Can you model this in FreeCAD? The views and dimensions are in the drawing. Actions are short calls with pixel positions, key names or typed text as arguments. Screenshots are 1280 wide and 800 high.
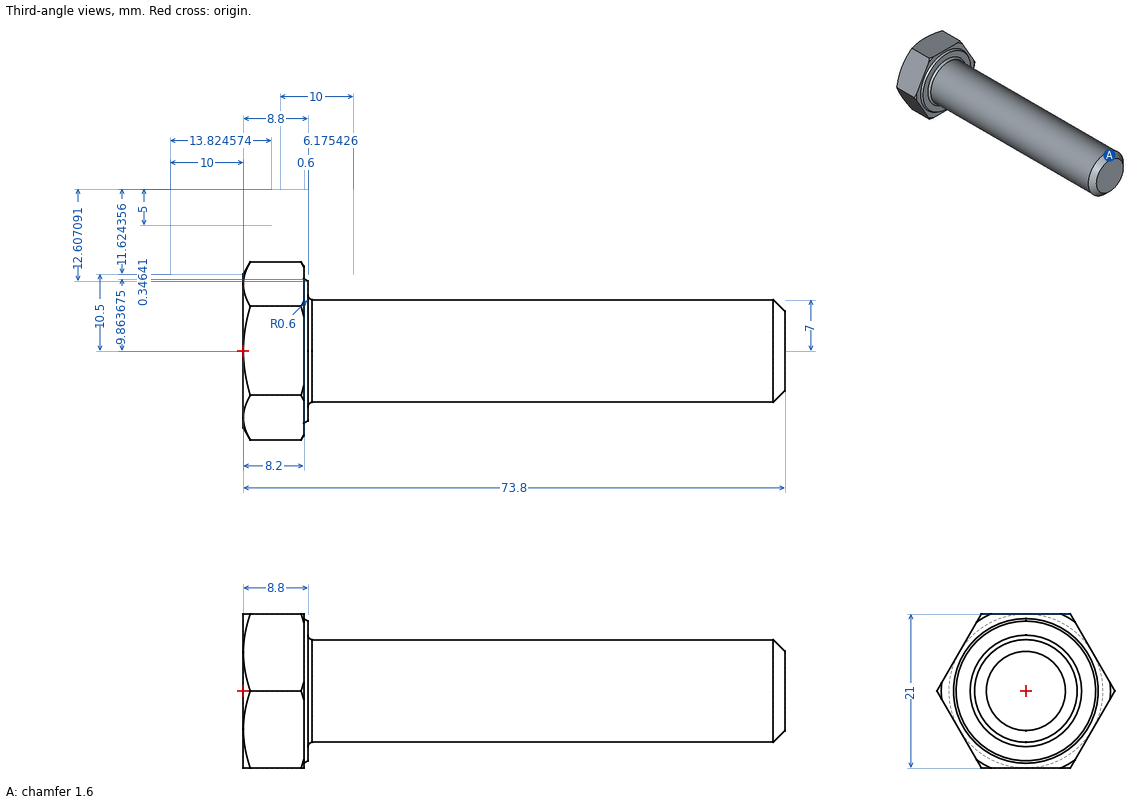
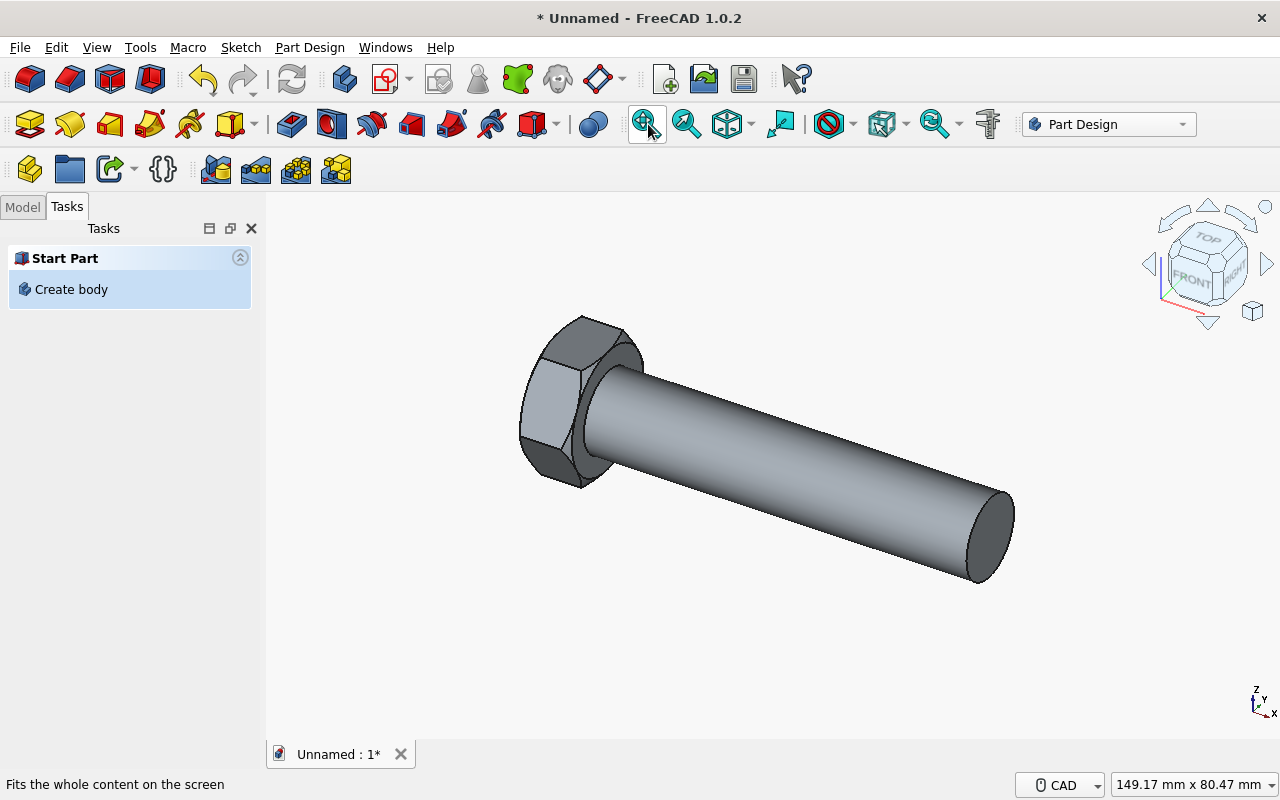
click(386, 80)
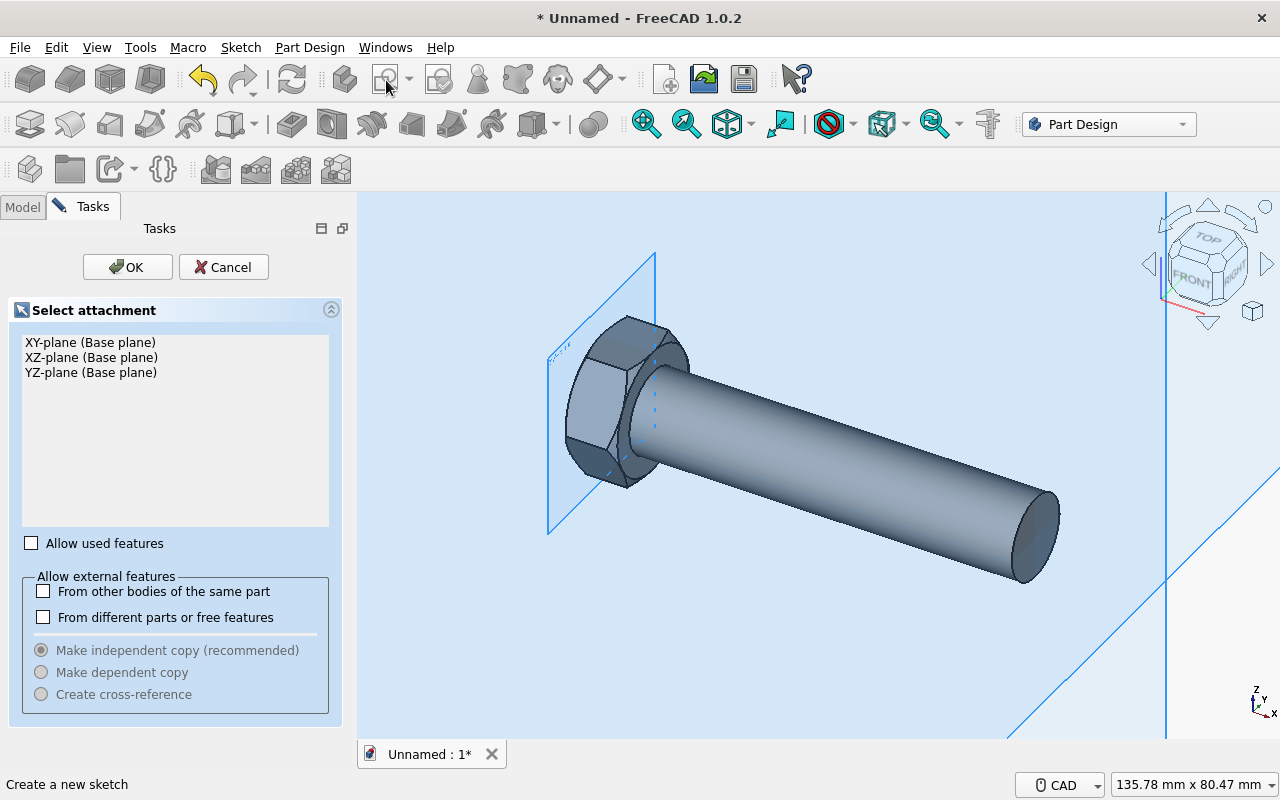
click(82, 342)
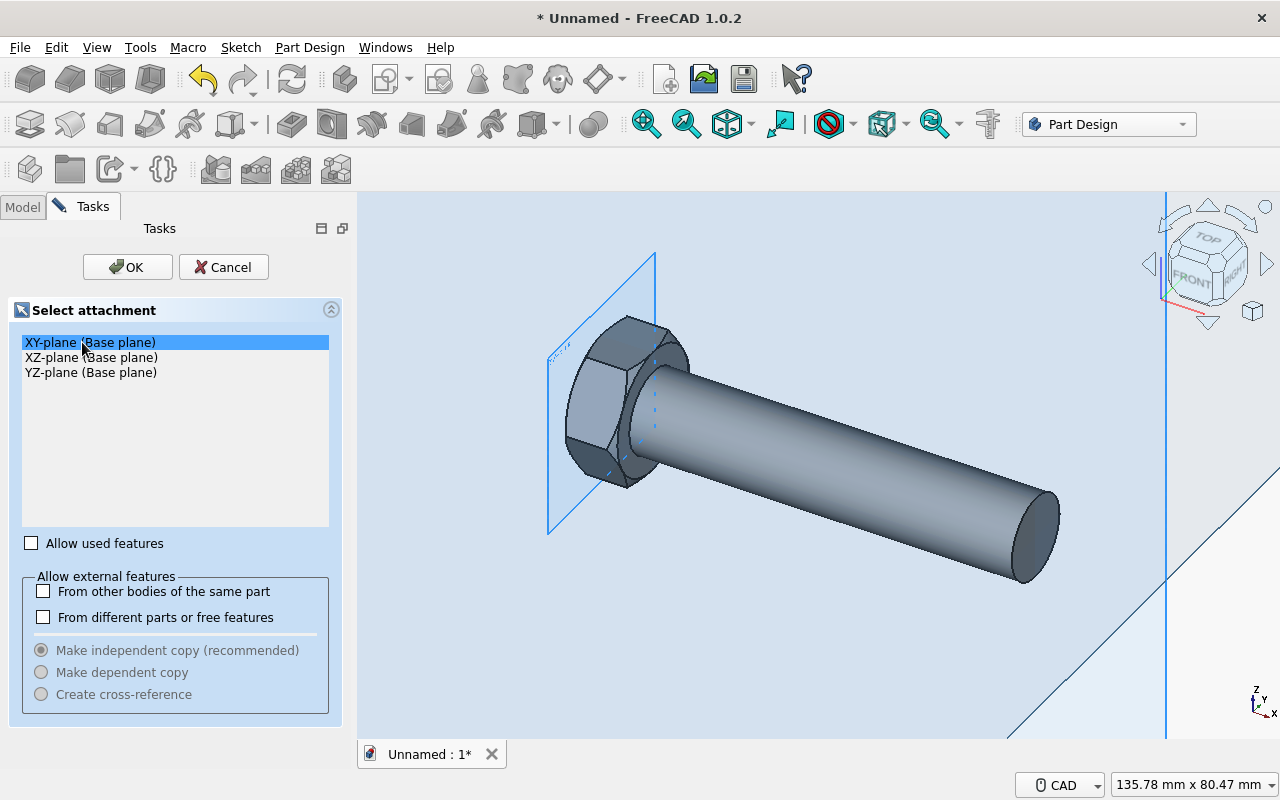
click(128, 267)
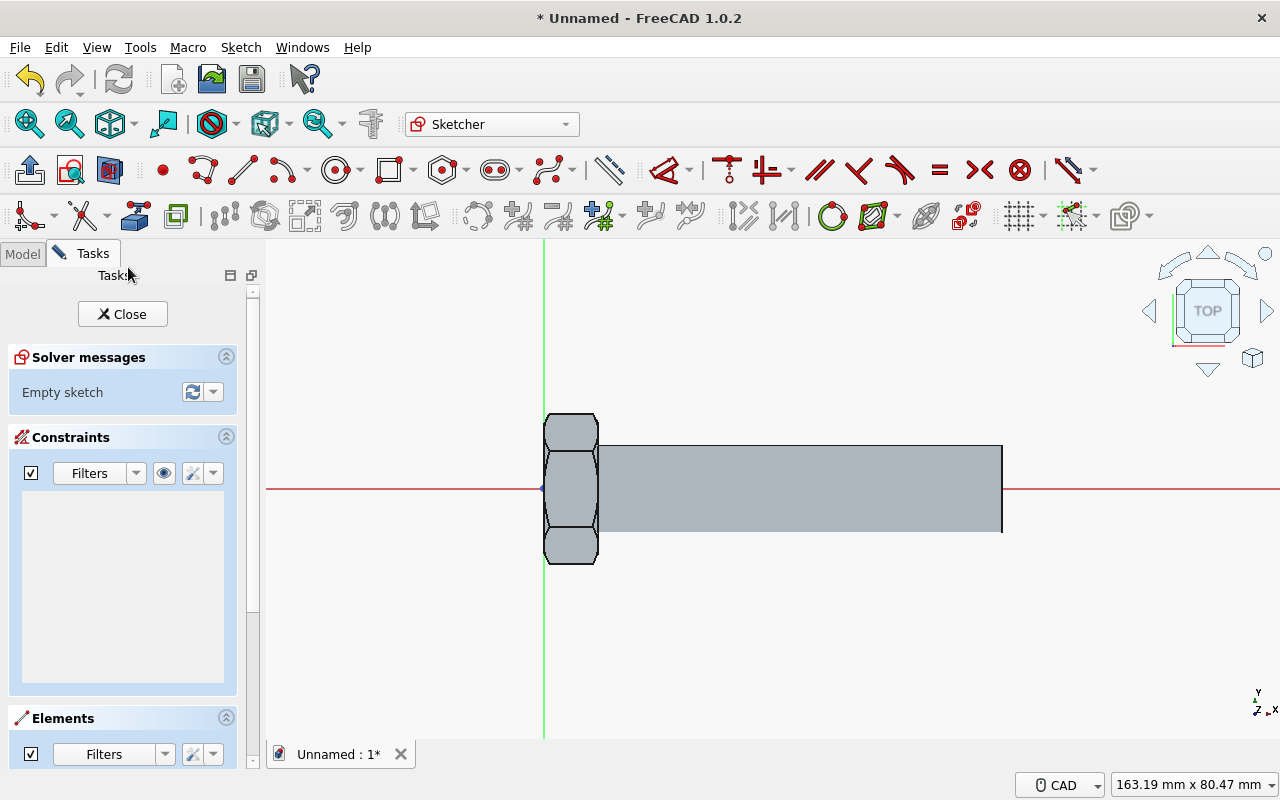
click(110, 170)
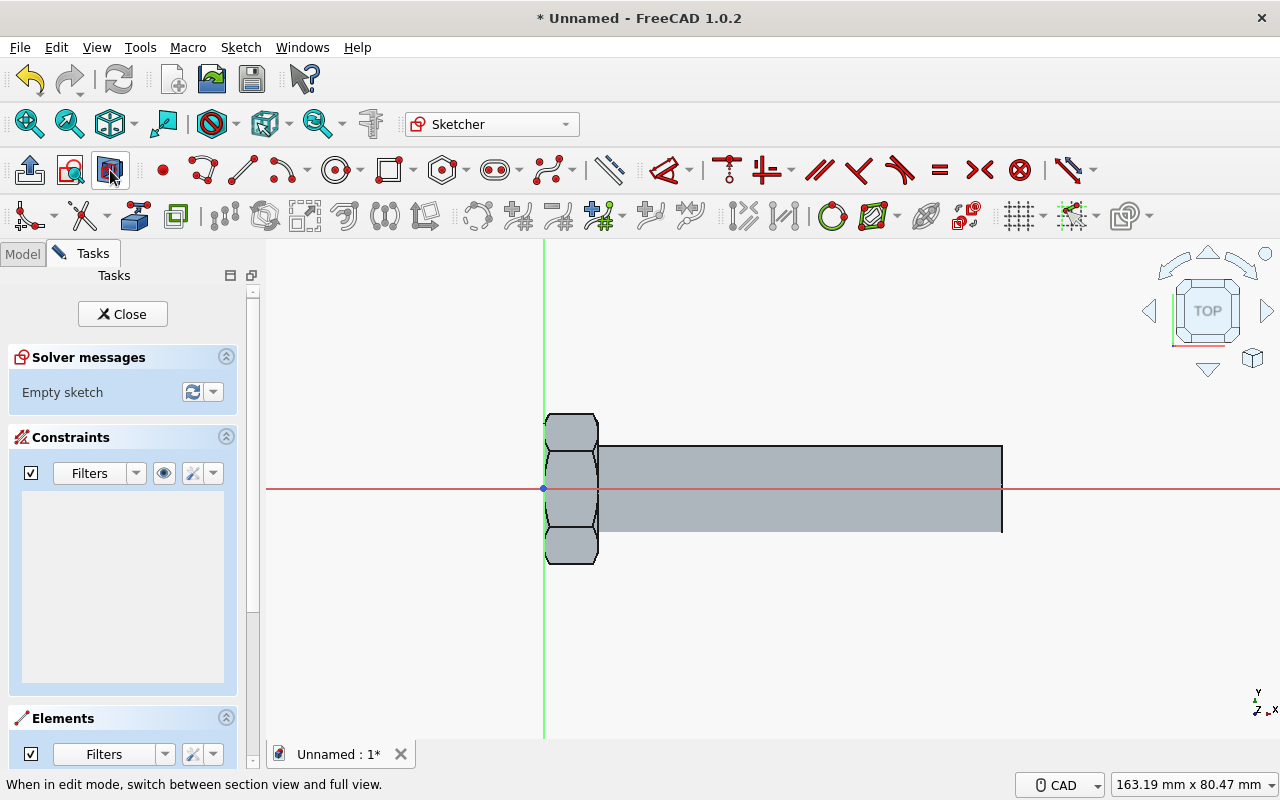
scroll(462, 364, up, 4)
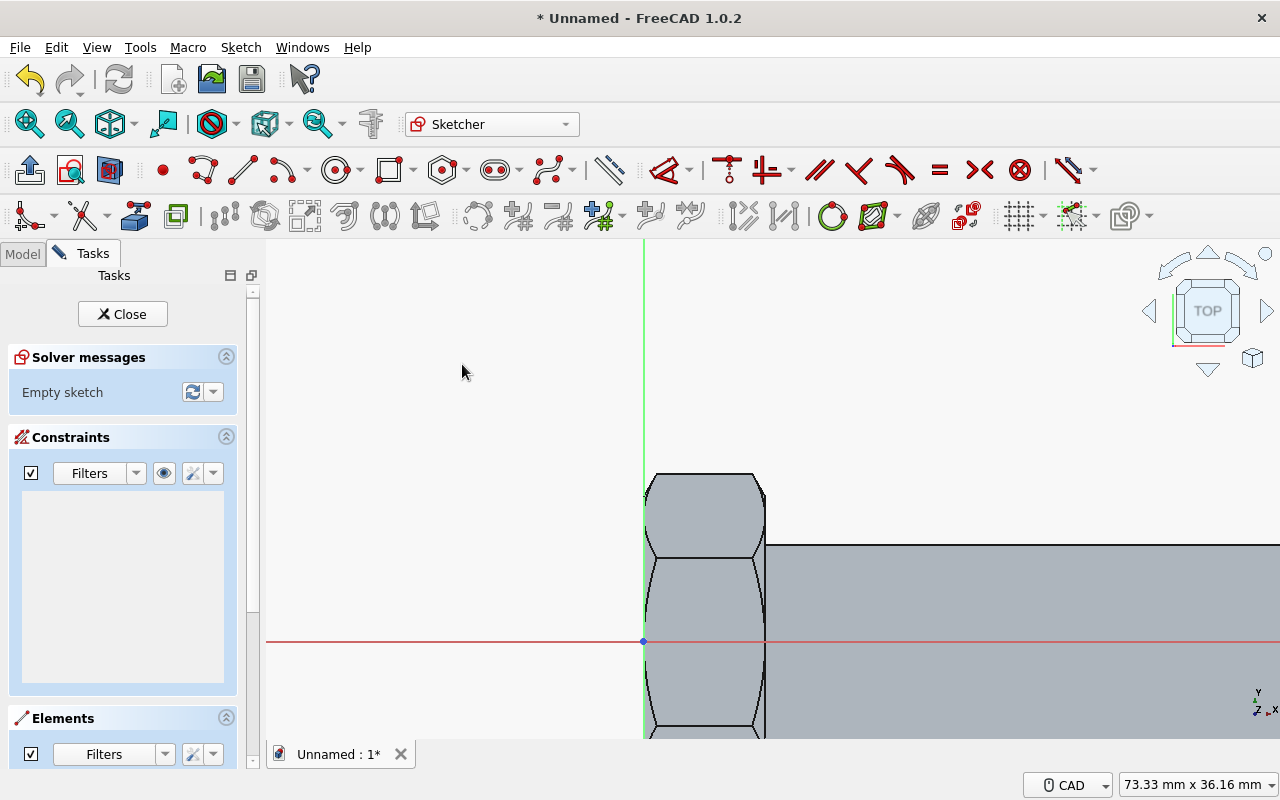
click(204, 170)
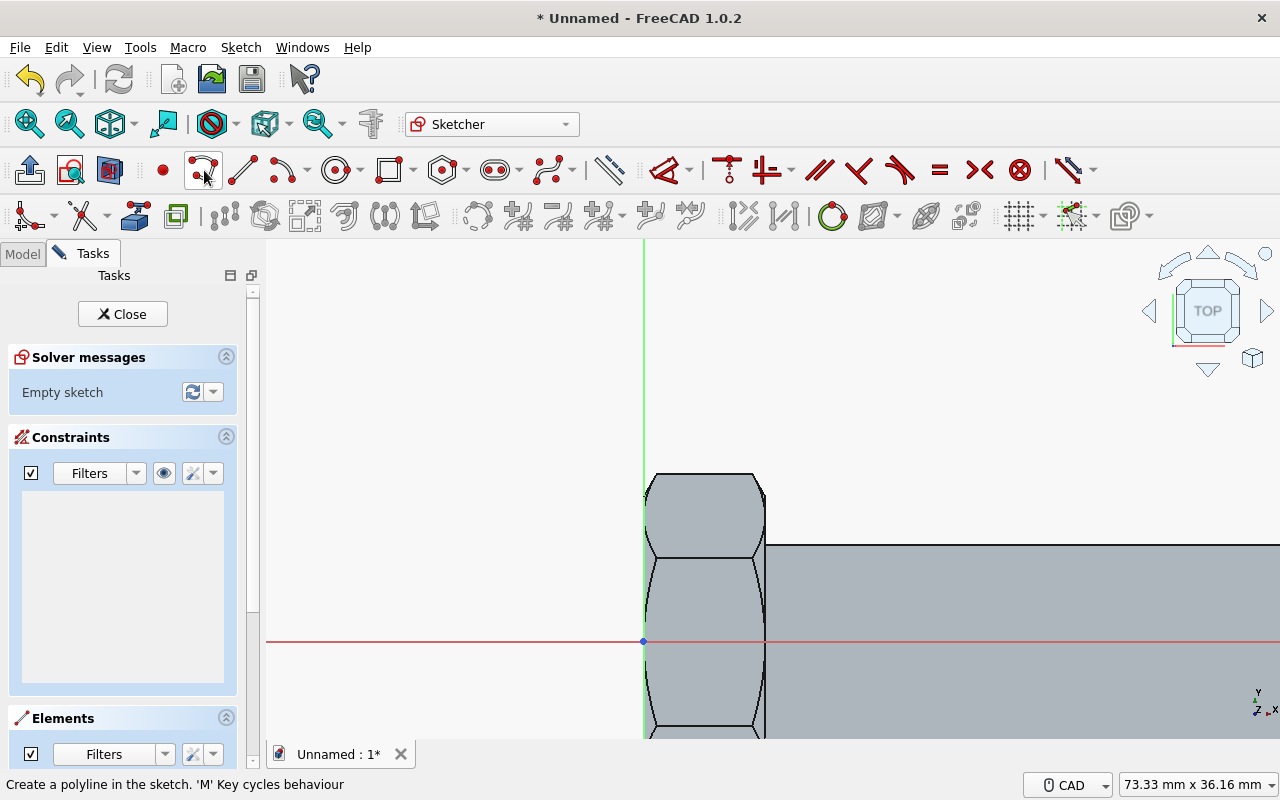
click(757, 505)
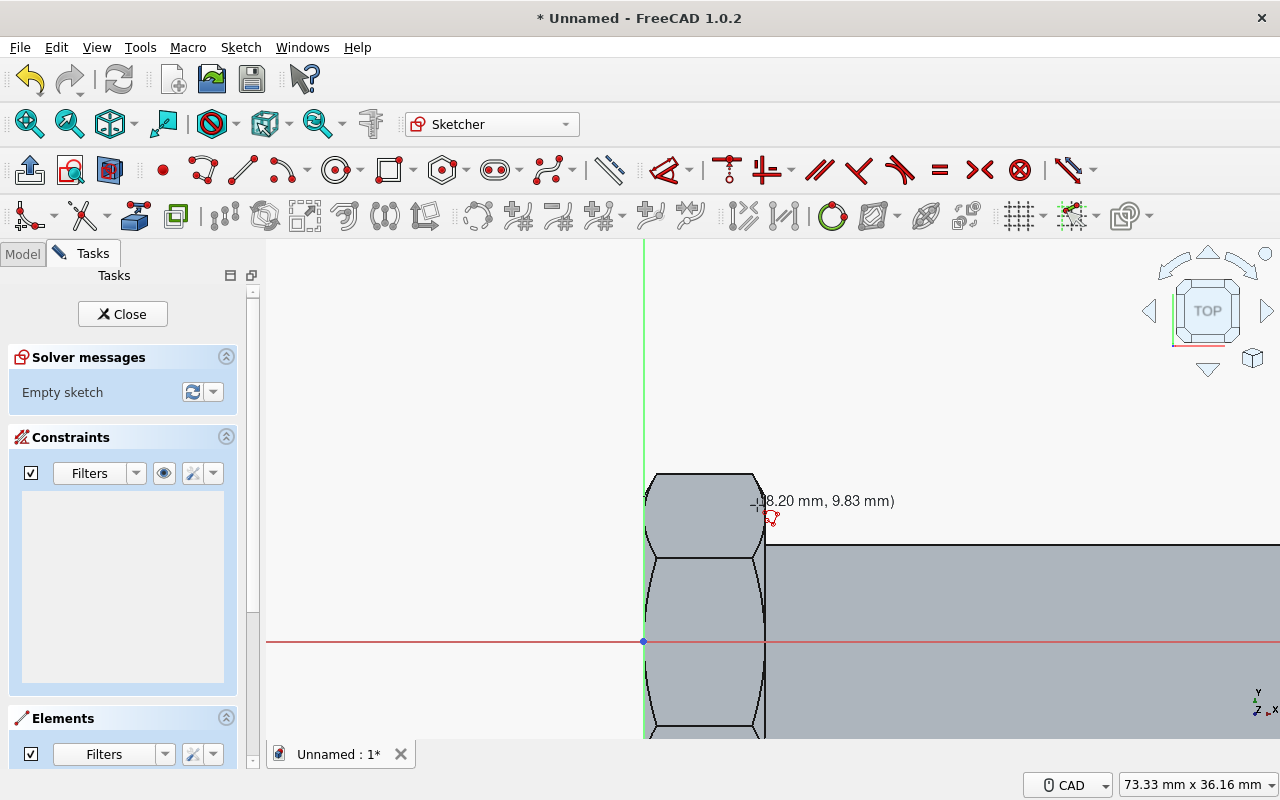
scroll(765, 510, up, 3)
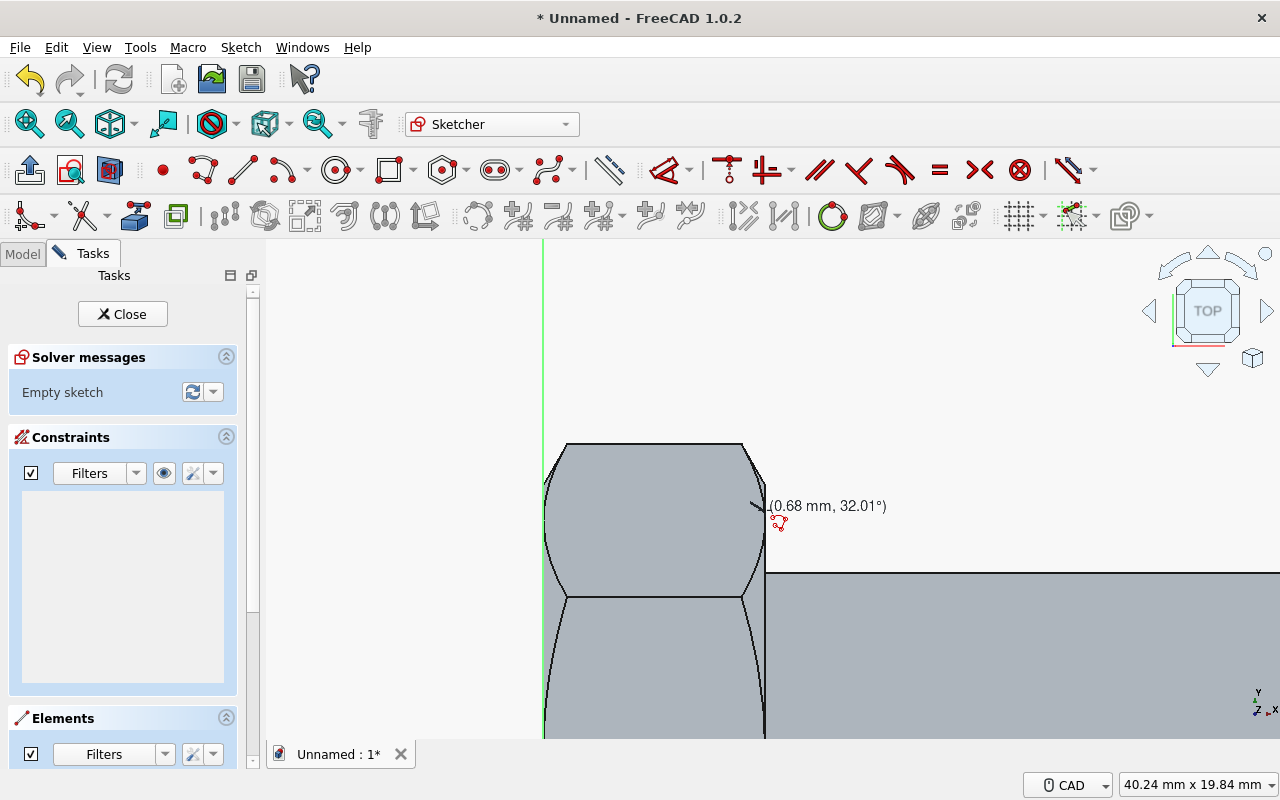
click(765, 510)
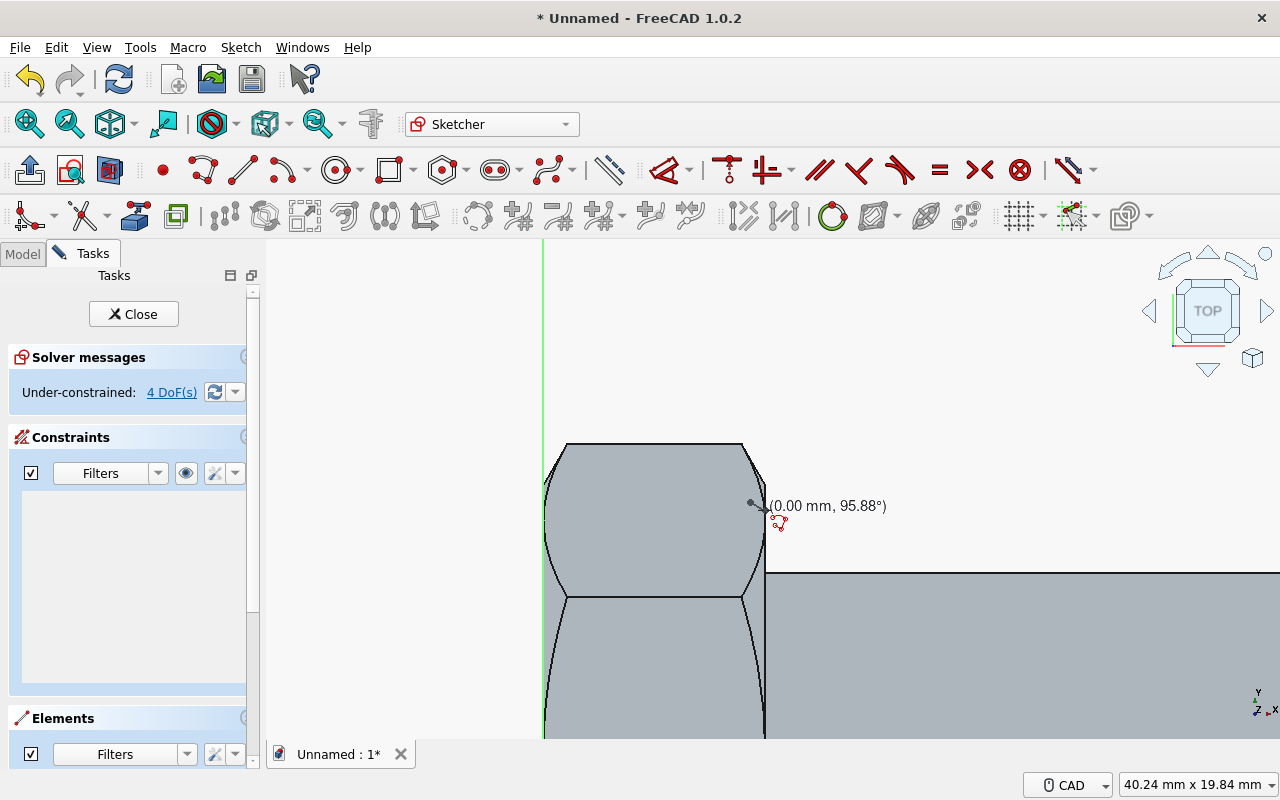
scroll(766, 511, down, 3)